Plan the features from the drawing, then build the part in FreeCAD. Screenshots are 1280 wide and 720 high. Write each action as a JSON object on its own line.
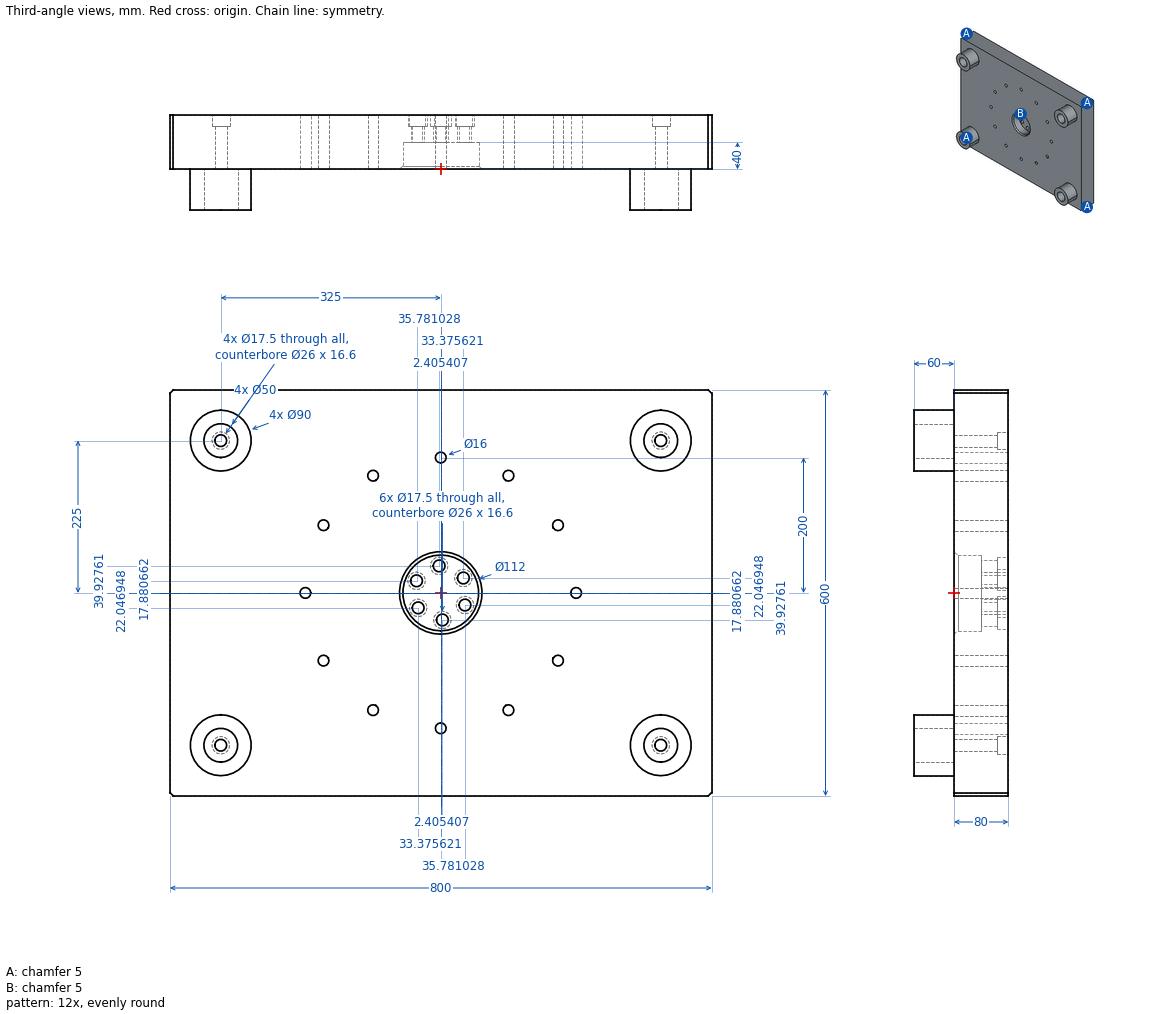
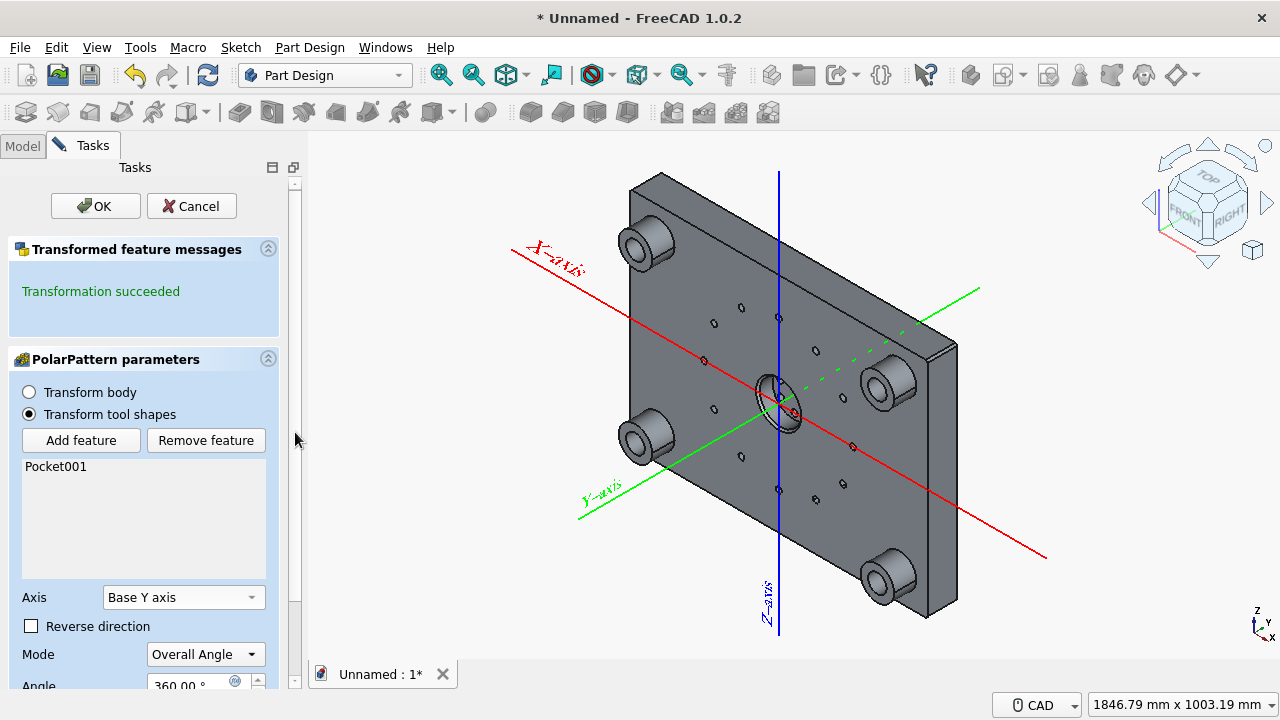
{"action": "left_click", "coordinate": [96, 206]}